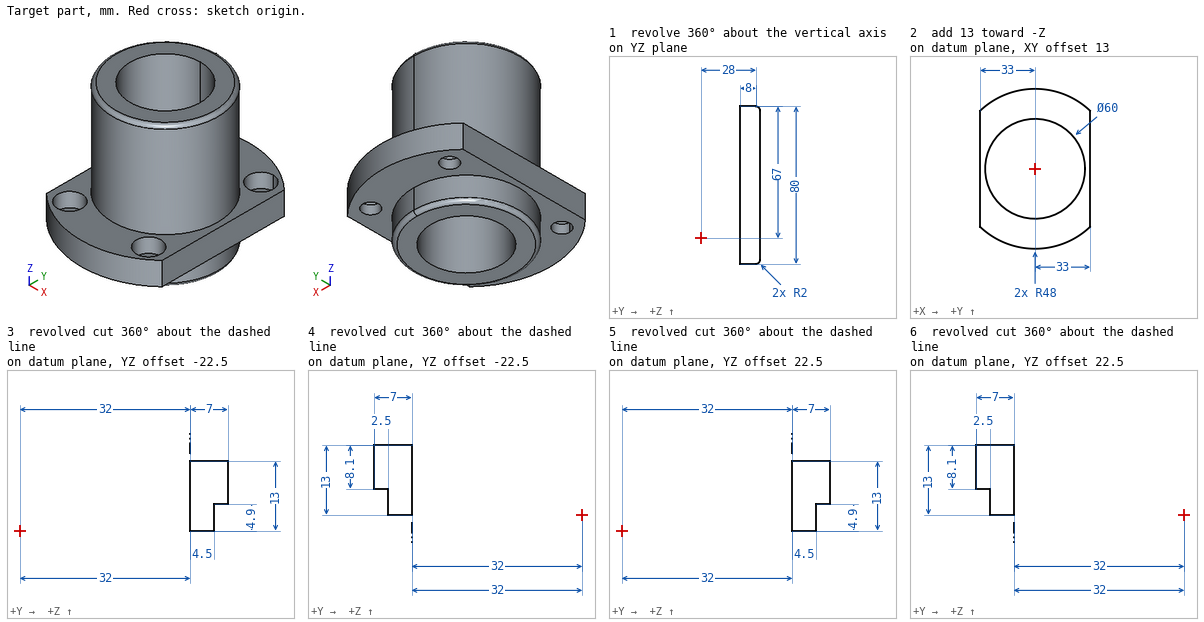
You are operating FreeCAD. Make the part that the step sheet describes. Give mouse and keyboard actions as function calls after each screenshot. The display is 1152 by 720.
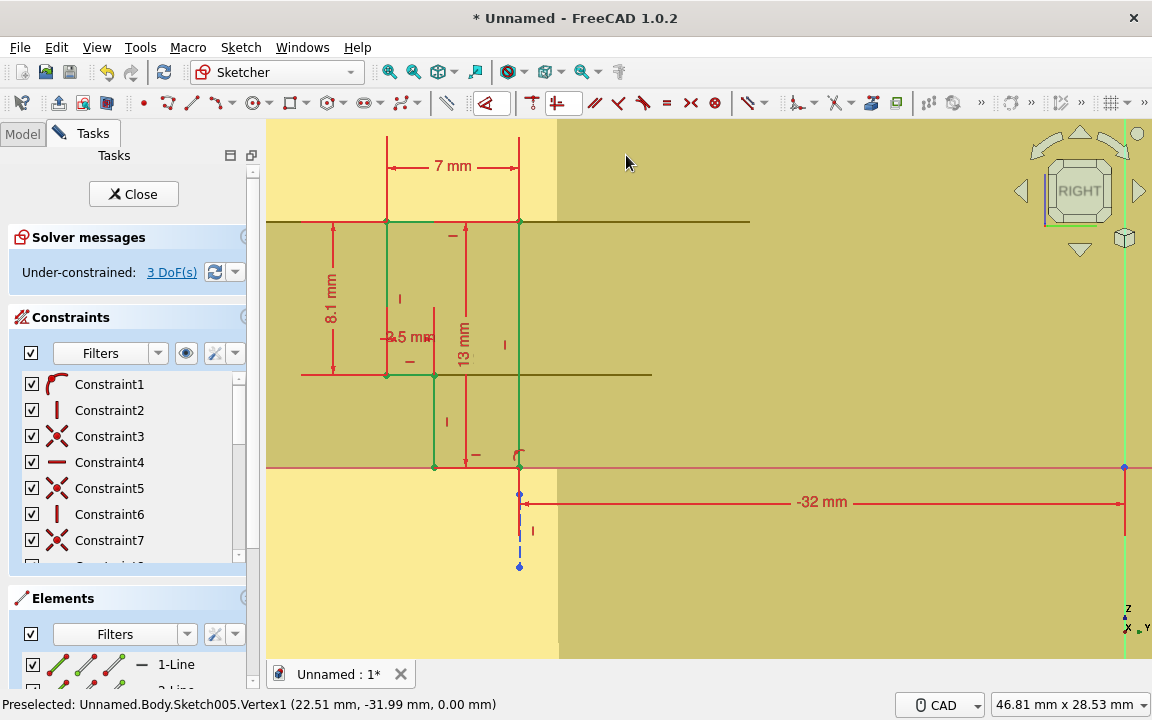
click(520, 494)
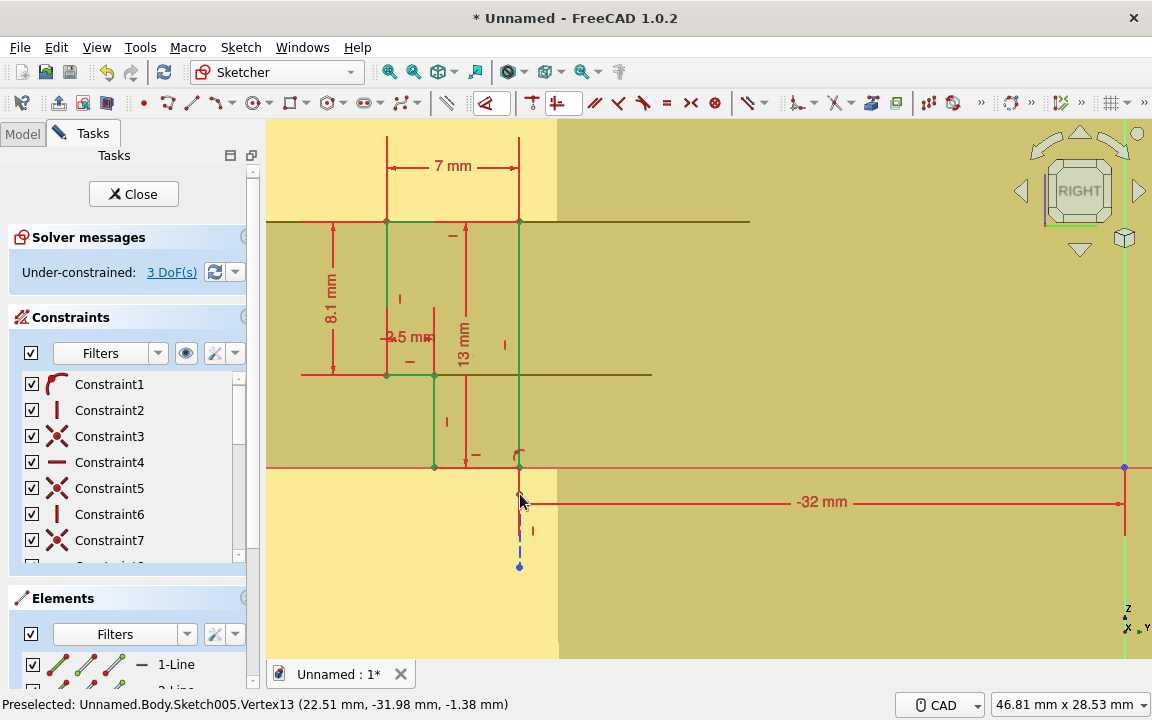
key(l)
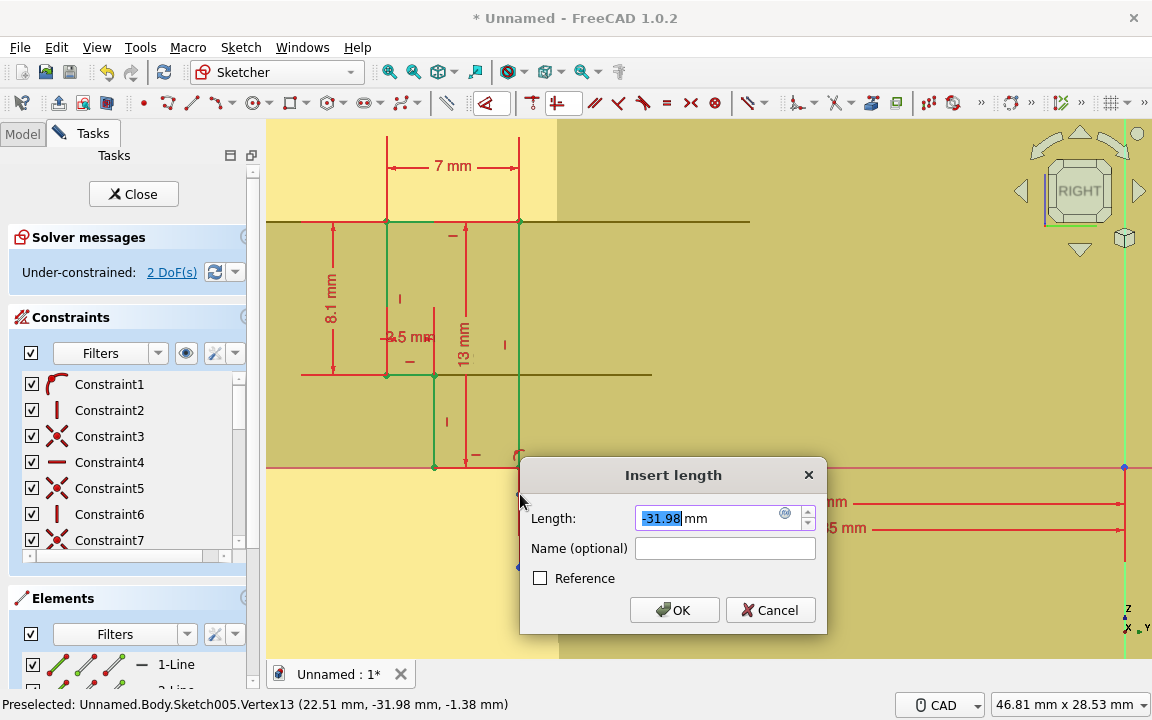
text(-32)
key(Return)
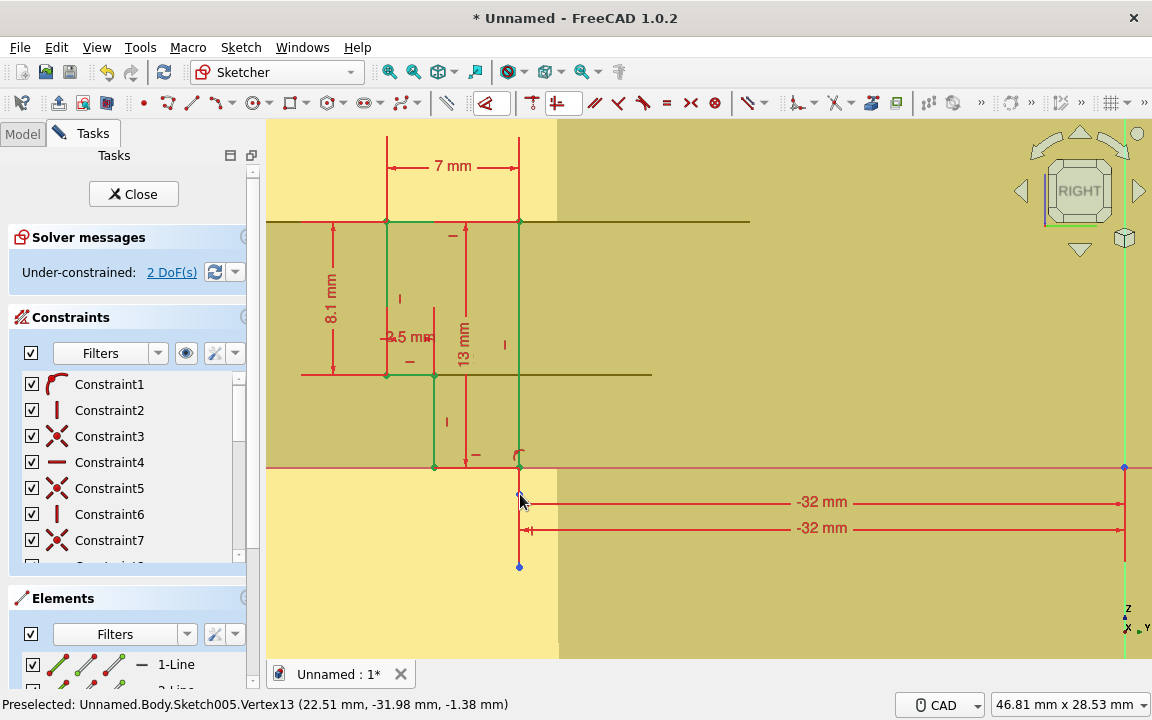
click(134, 194)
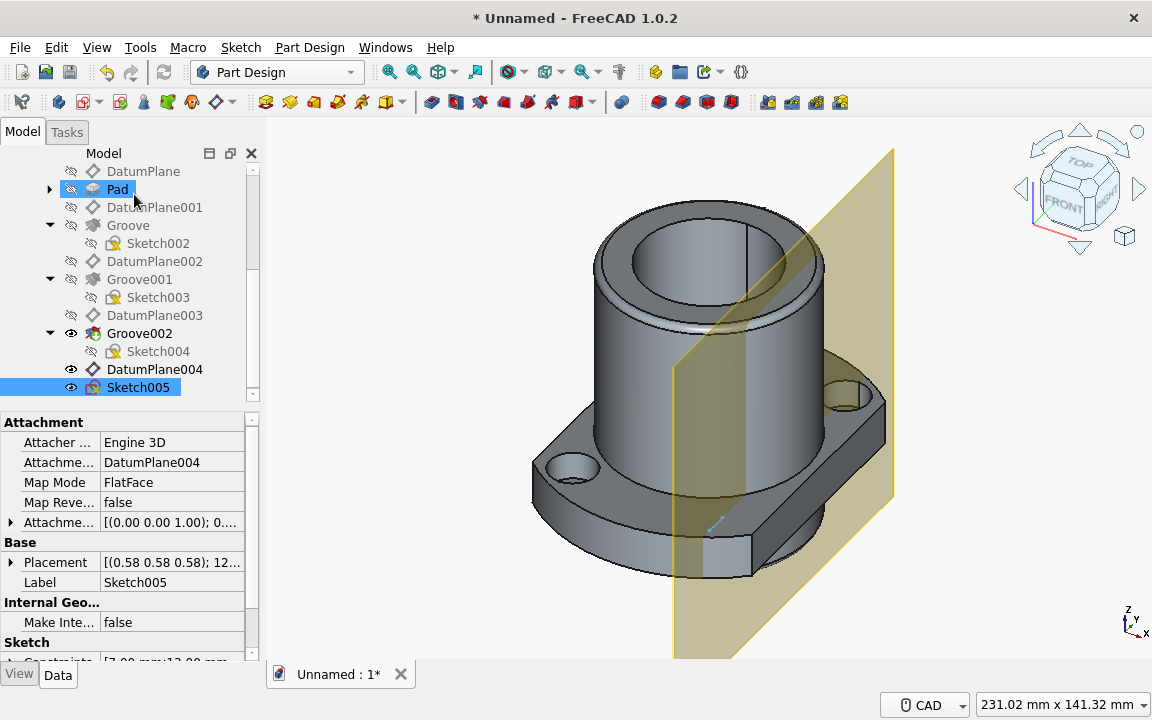
click(480, 102)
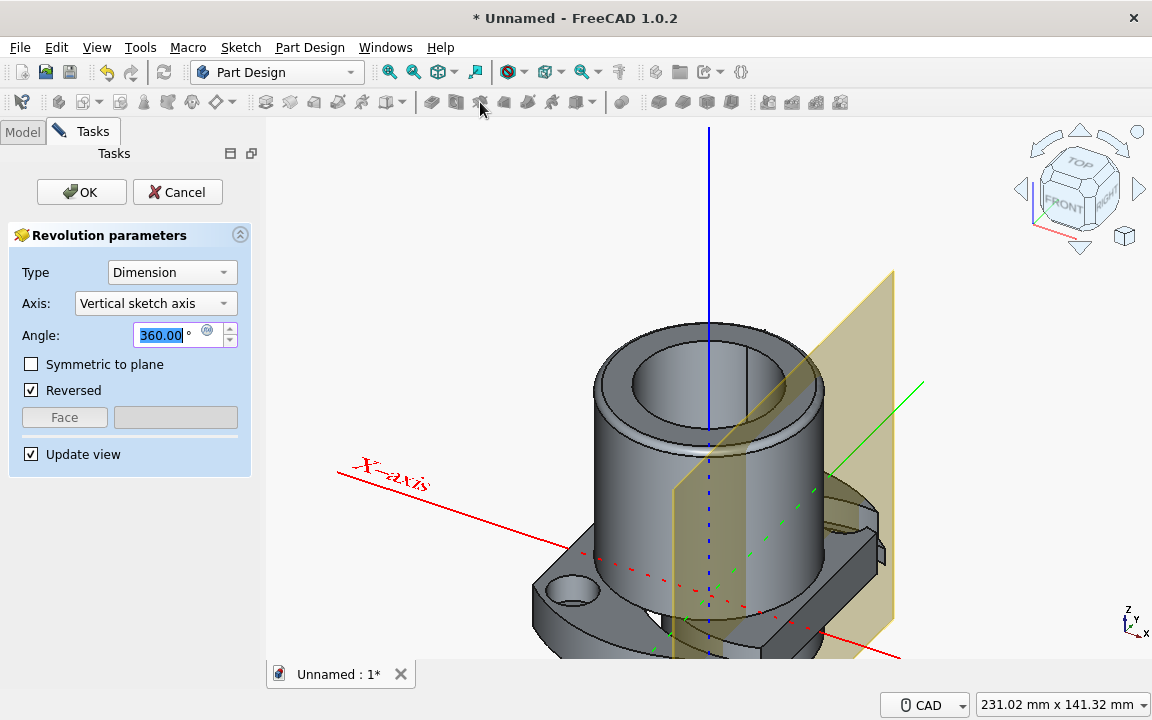
click(156, 304)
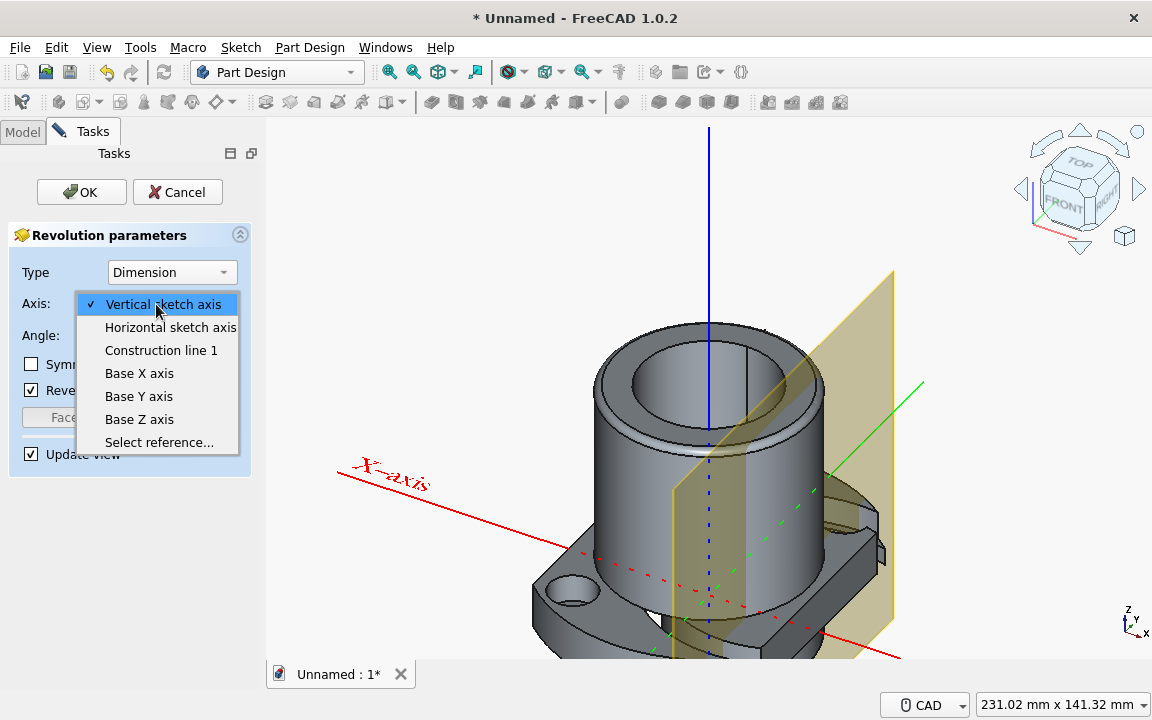
click(156, 350)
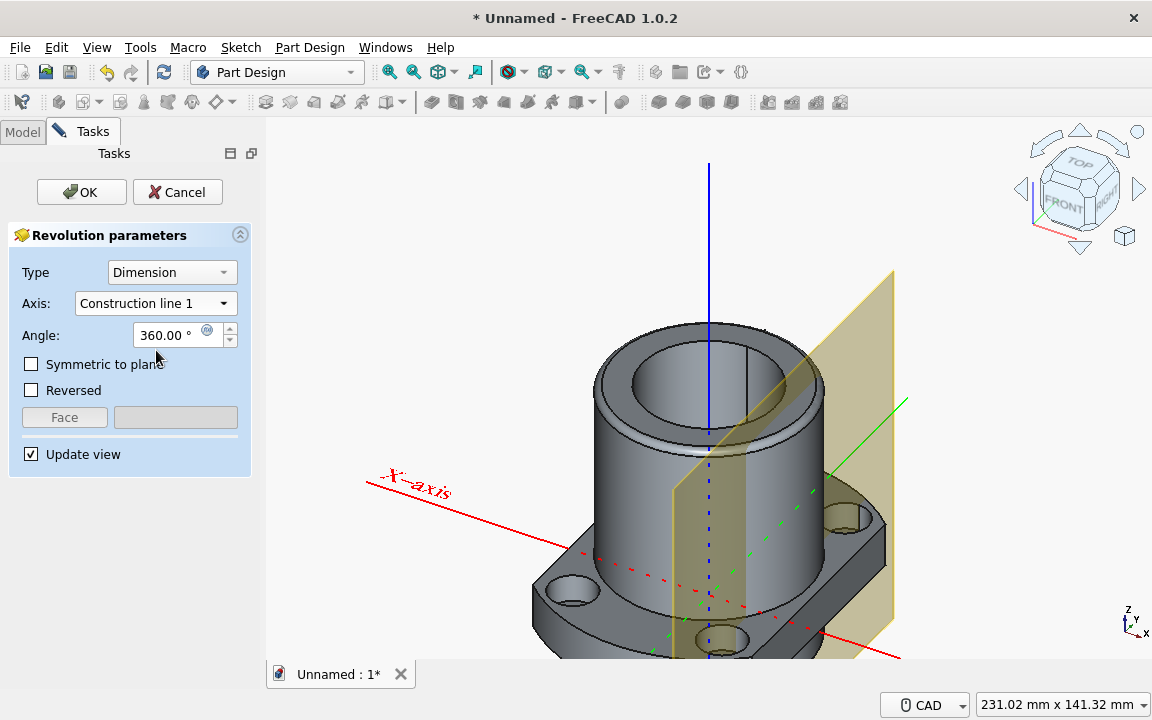
click(82, 192)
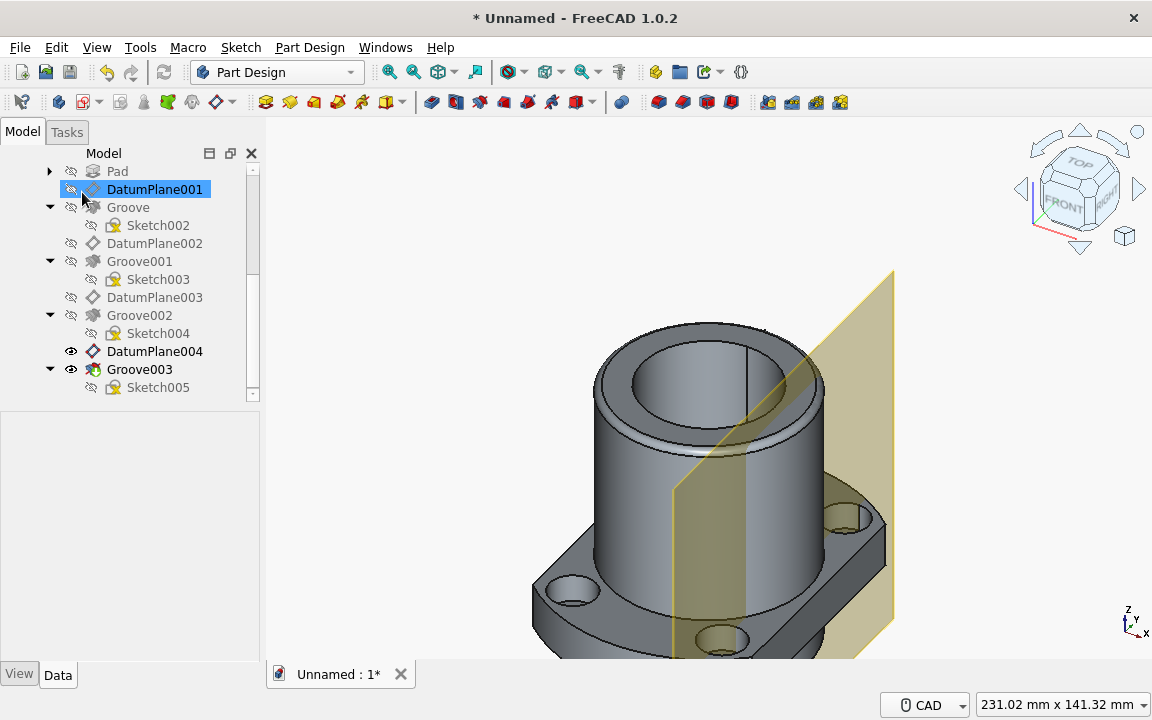
click(116, 351)
key(space)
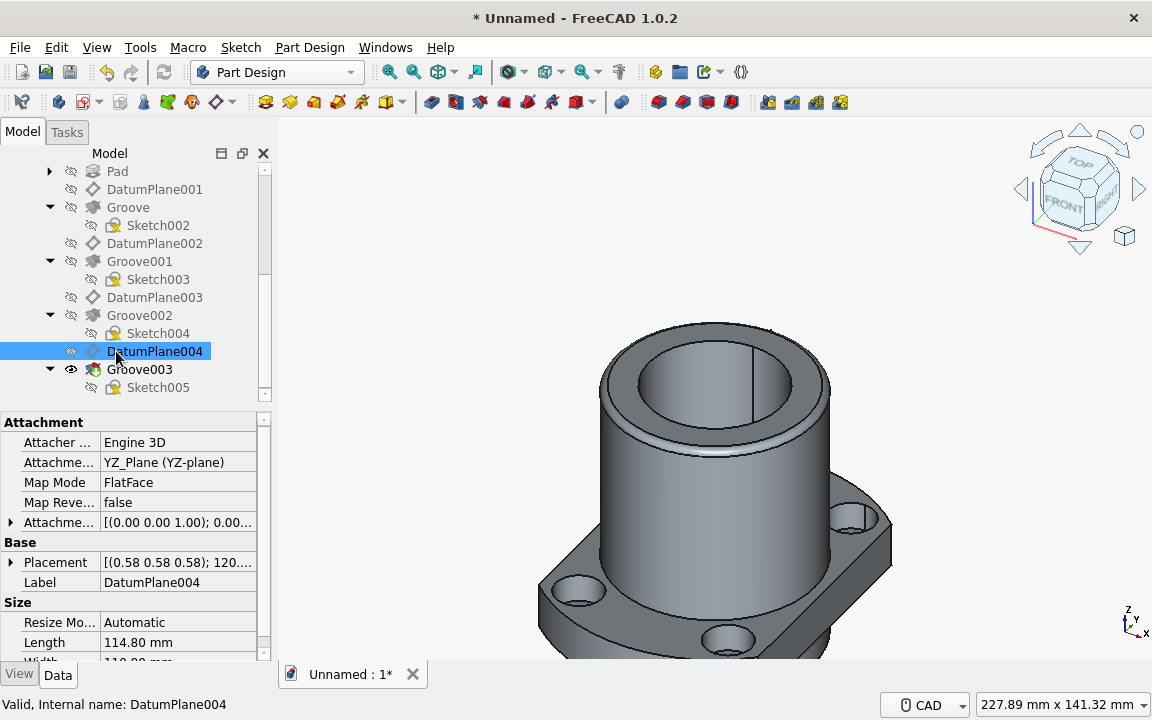
key(0)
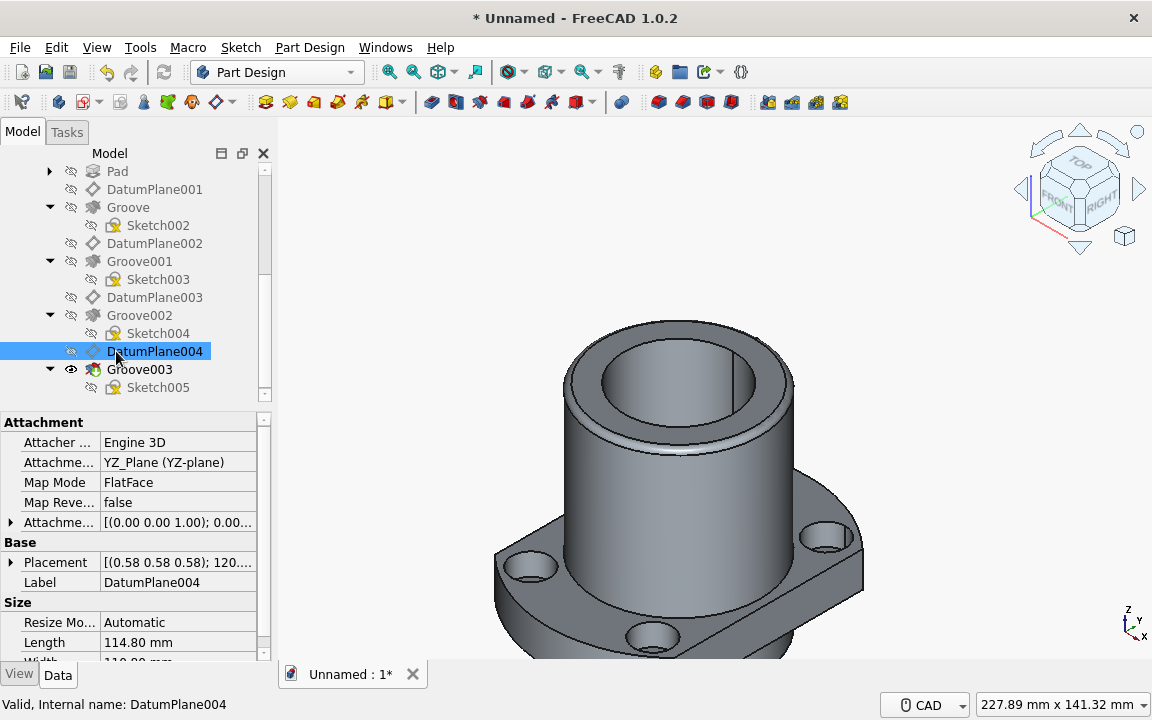
click(390, 72)